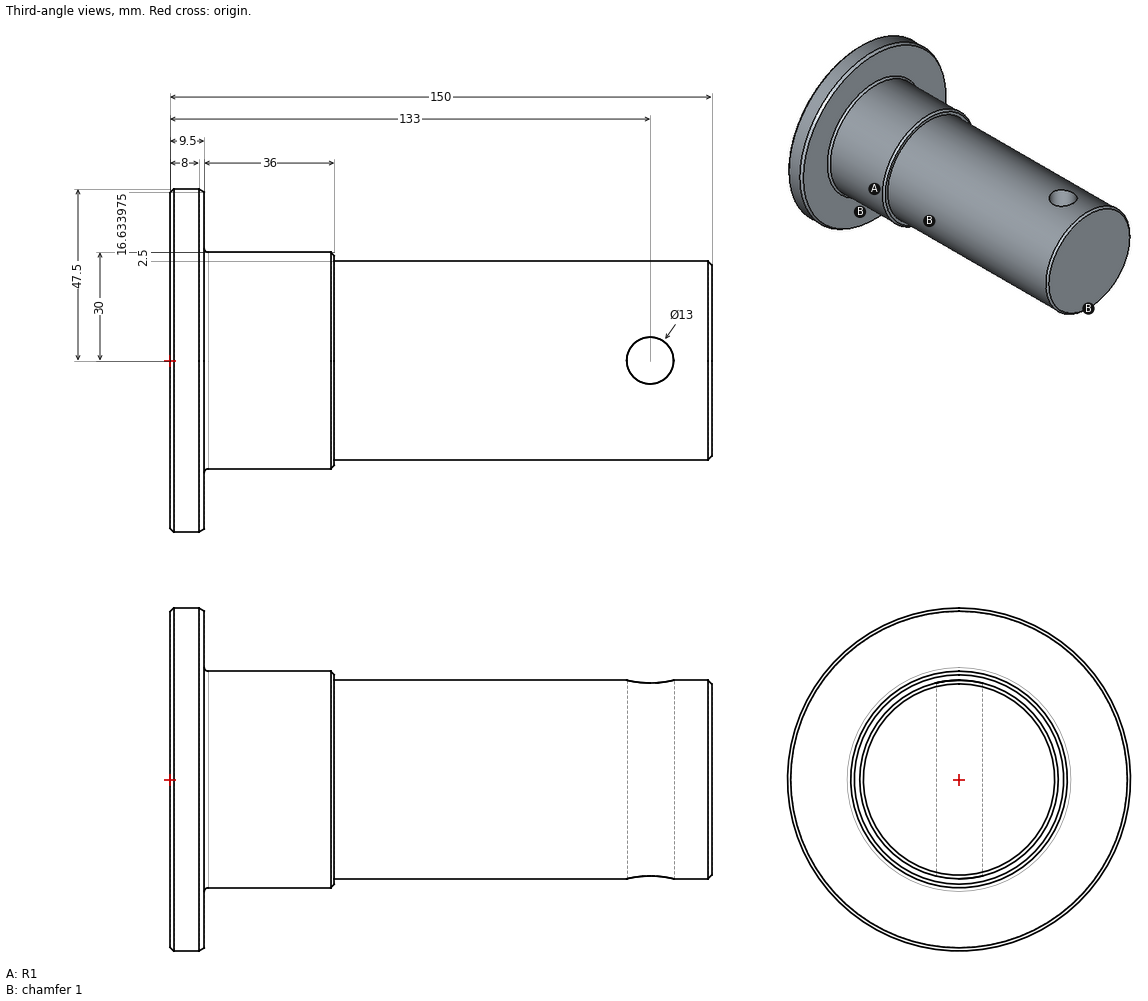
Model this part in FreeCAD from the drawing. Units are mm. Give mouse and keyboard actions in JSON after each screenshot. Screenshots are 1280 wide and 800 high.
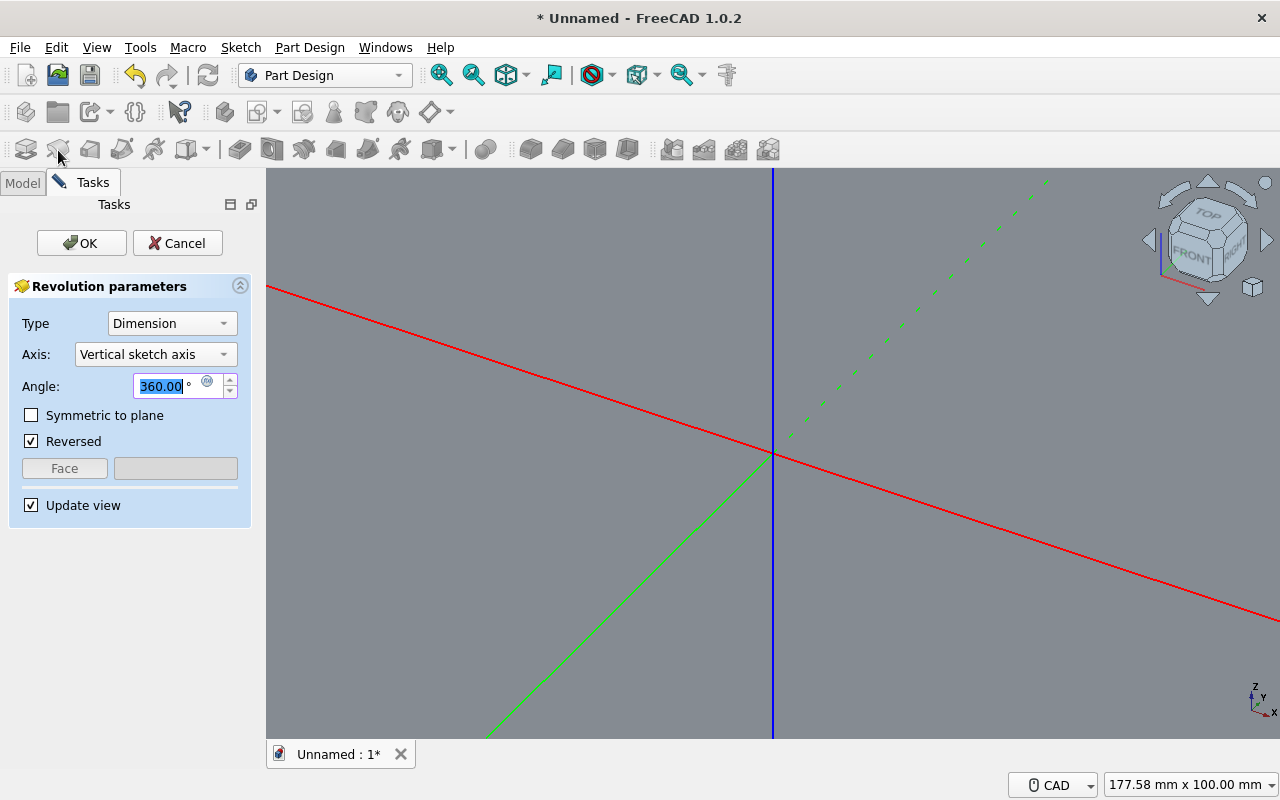
{"action": "left_click", "coordinate": [156, 354]}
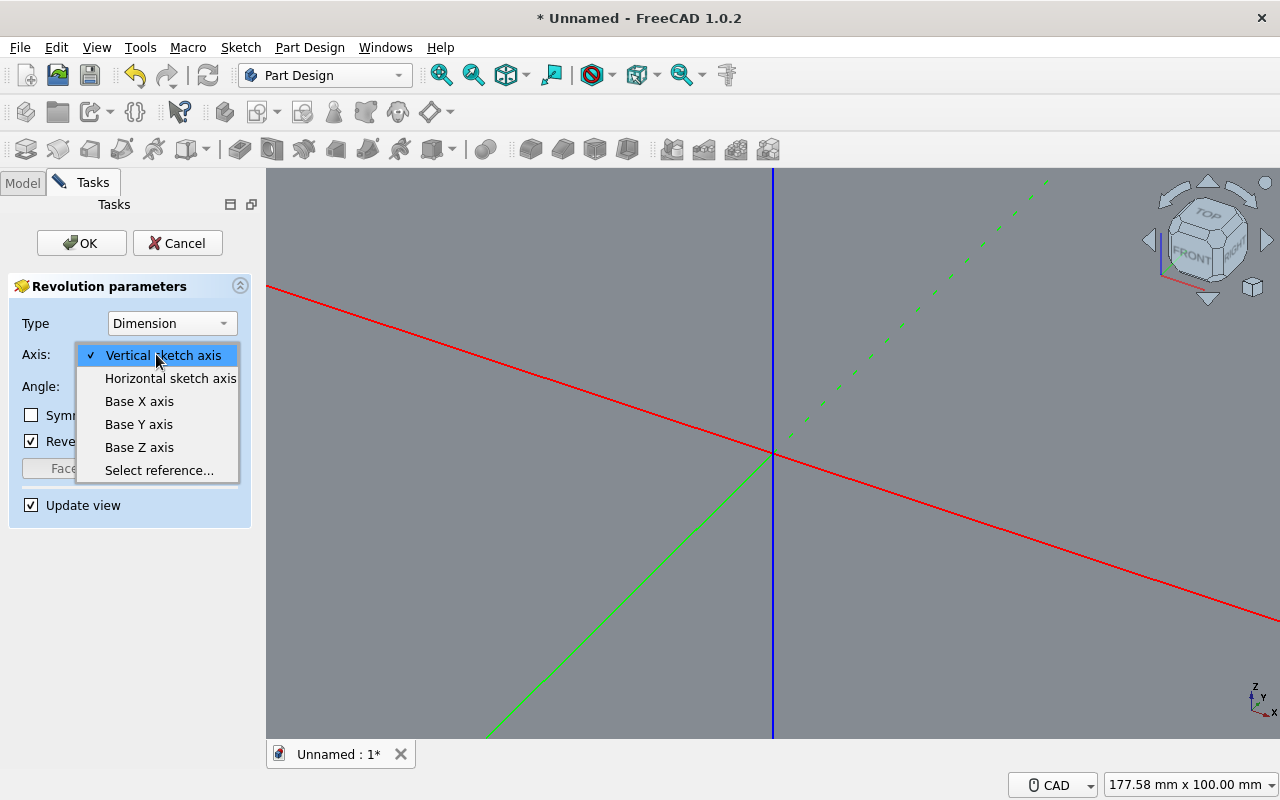
{"action": "left_click", "coordinate": [156, 378]}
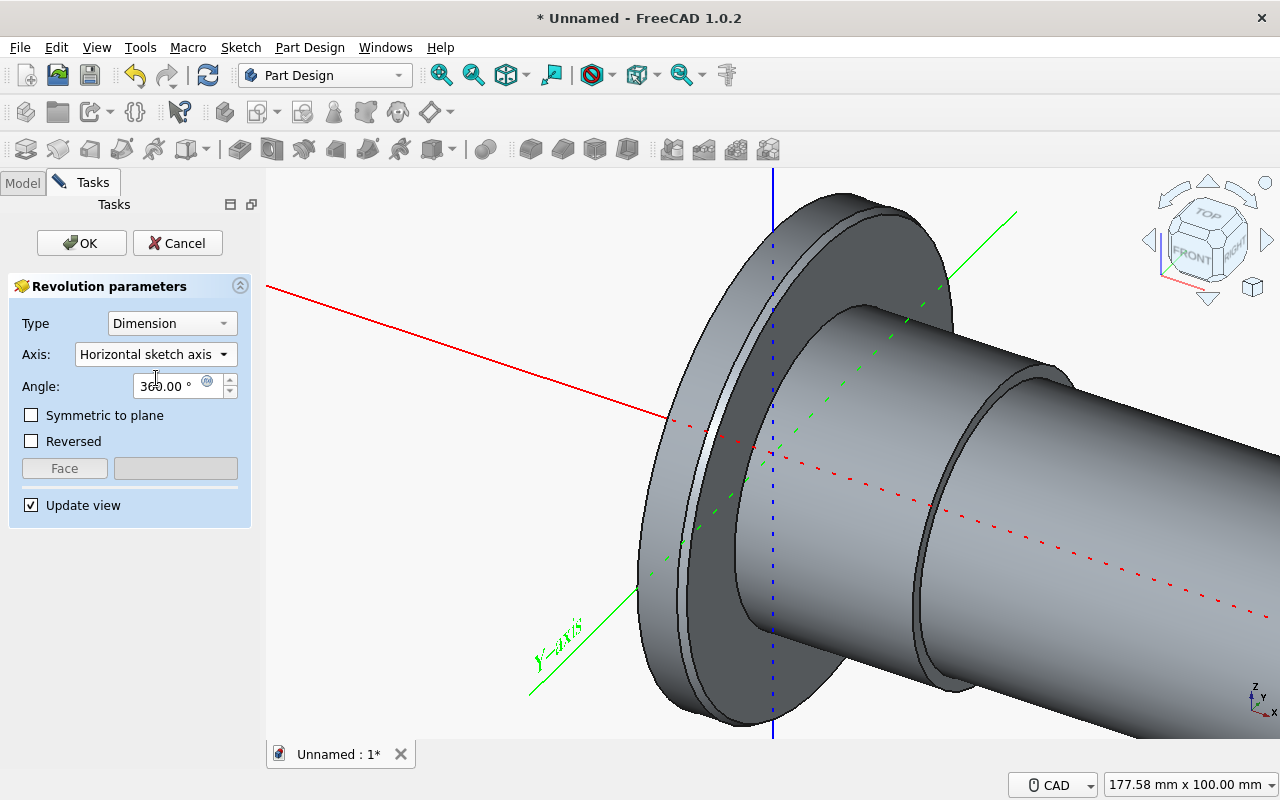
{"action": "left_click", "coordinate": [82, 243]}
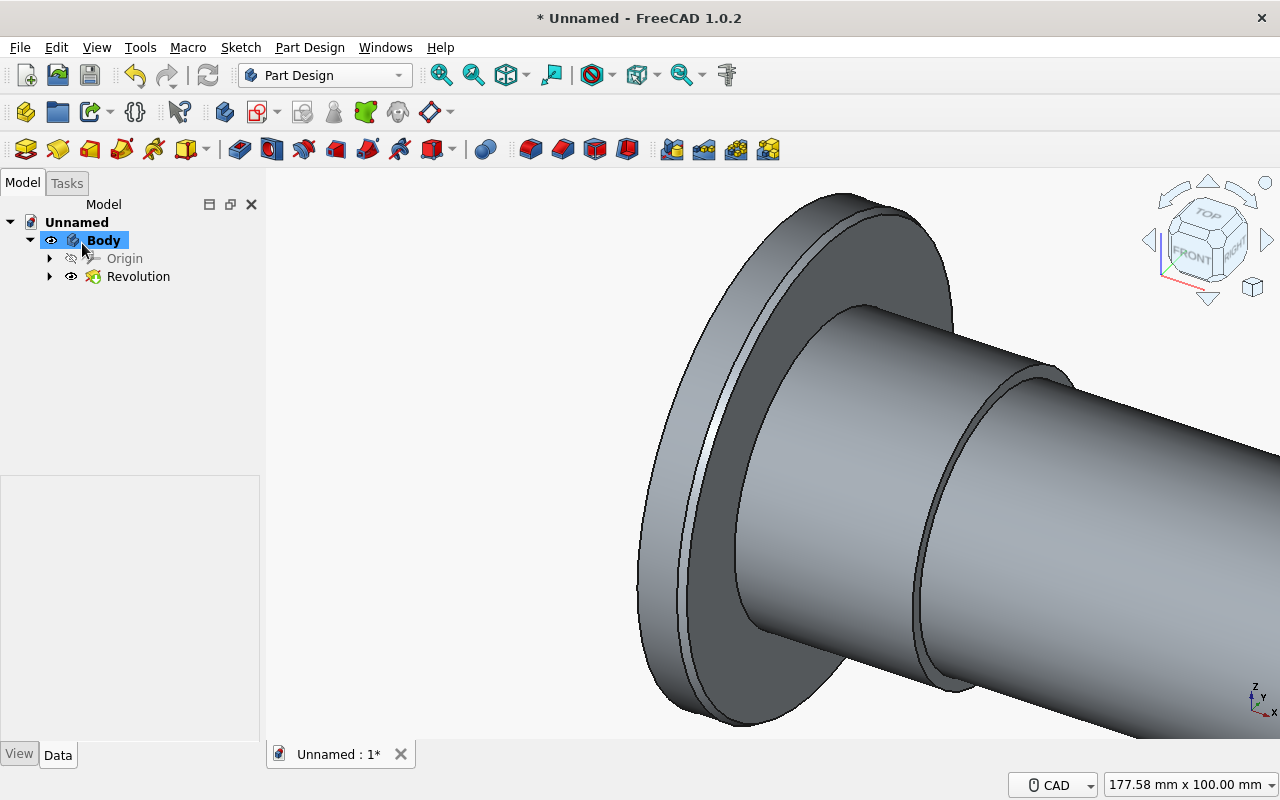
{"action": "key", "text": "v f"}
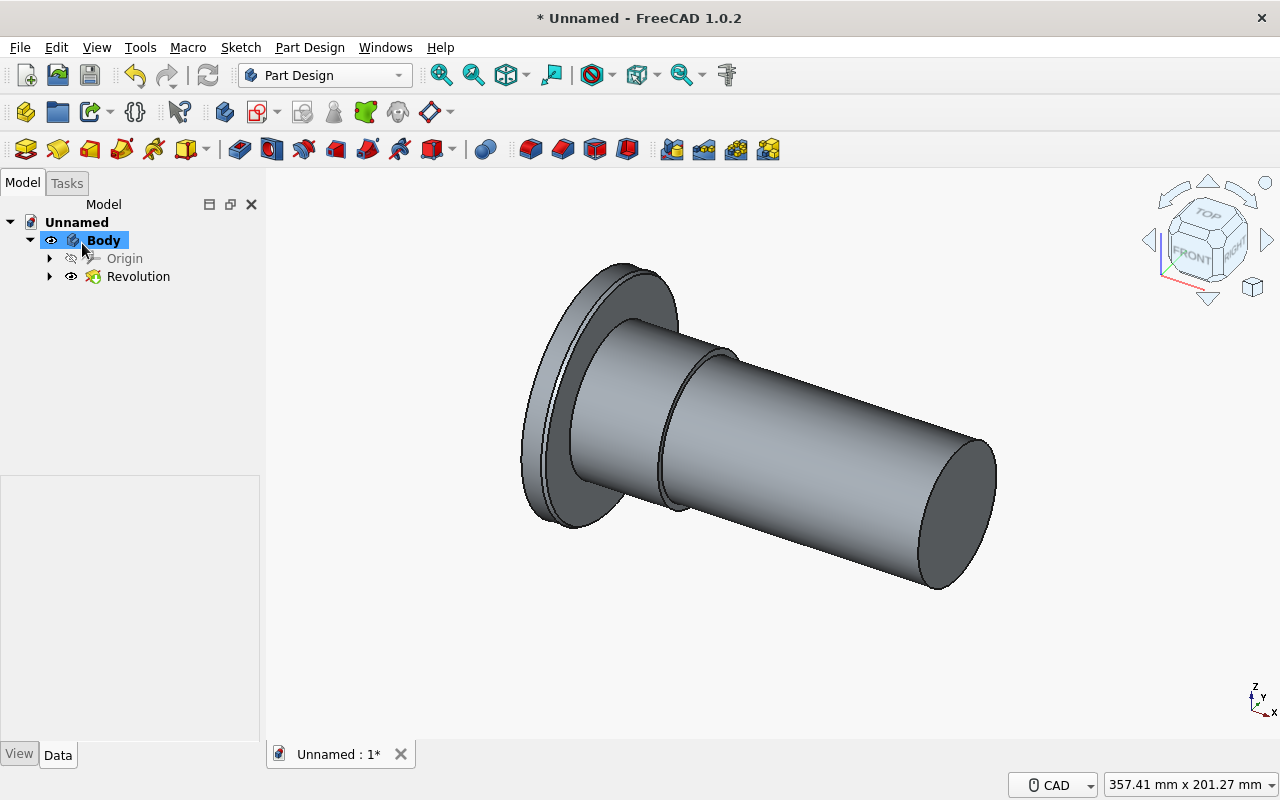
{"action": "key", "text": "0"}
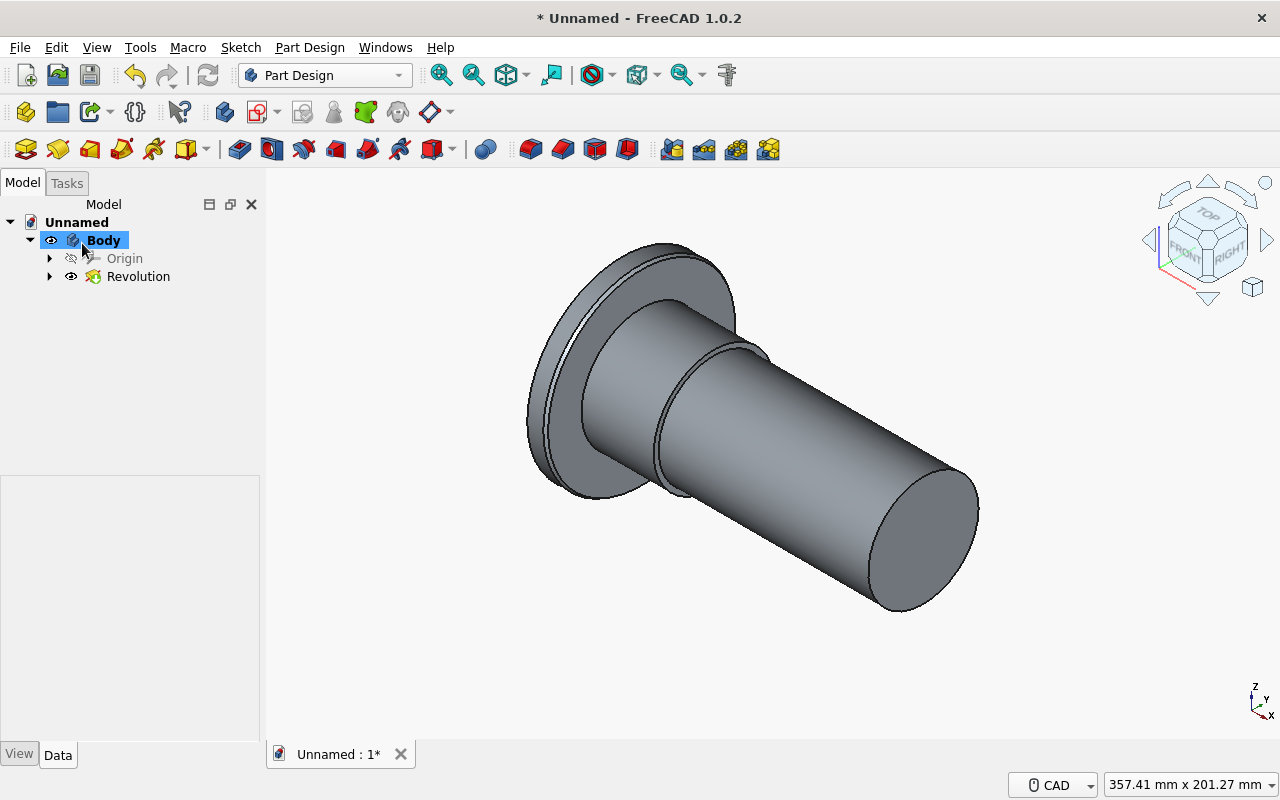
{"action": "key", "text": "2"}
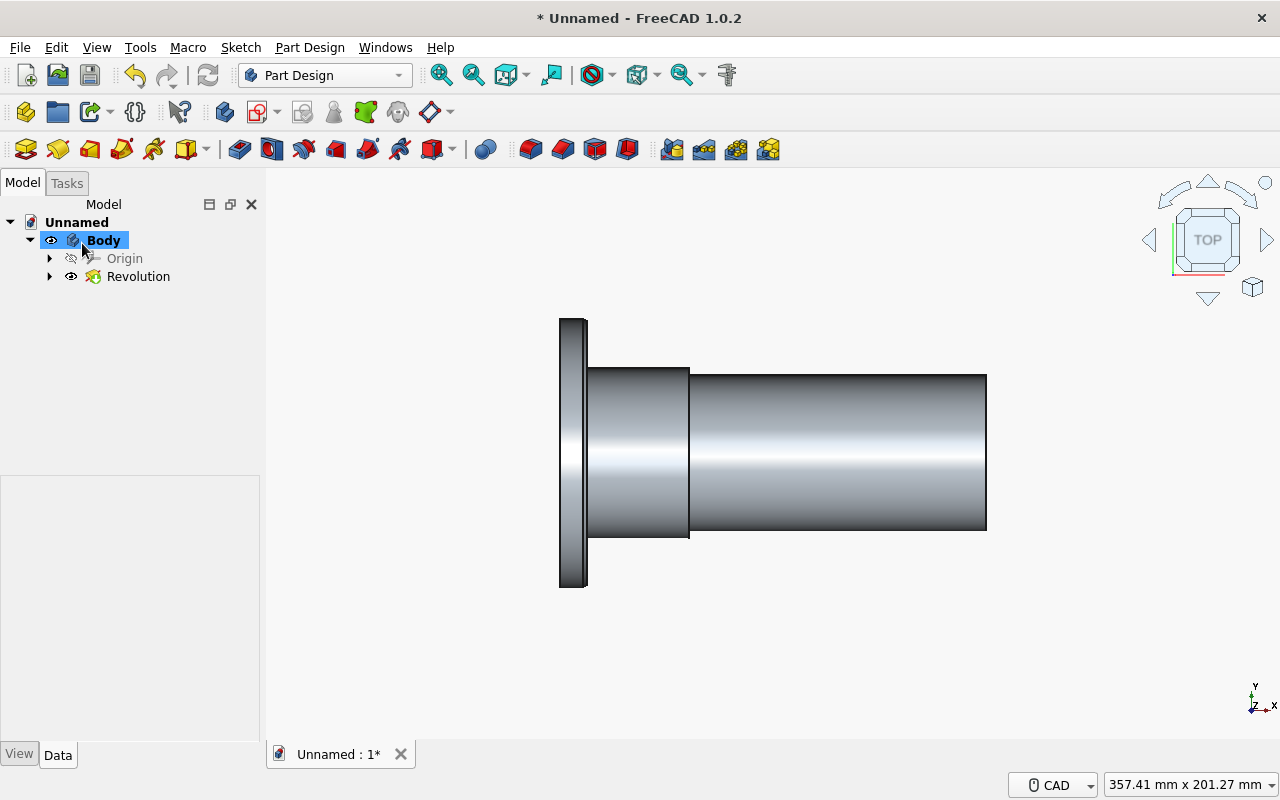
{"action": "key", "text": "1"}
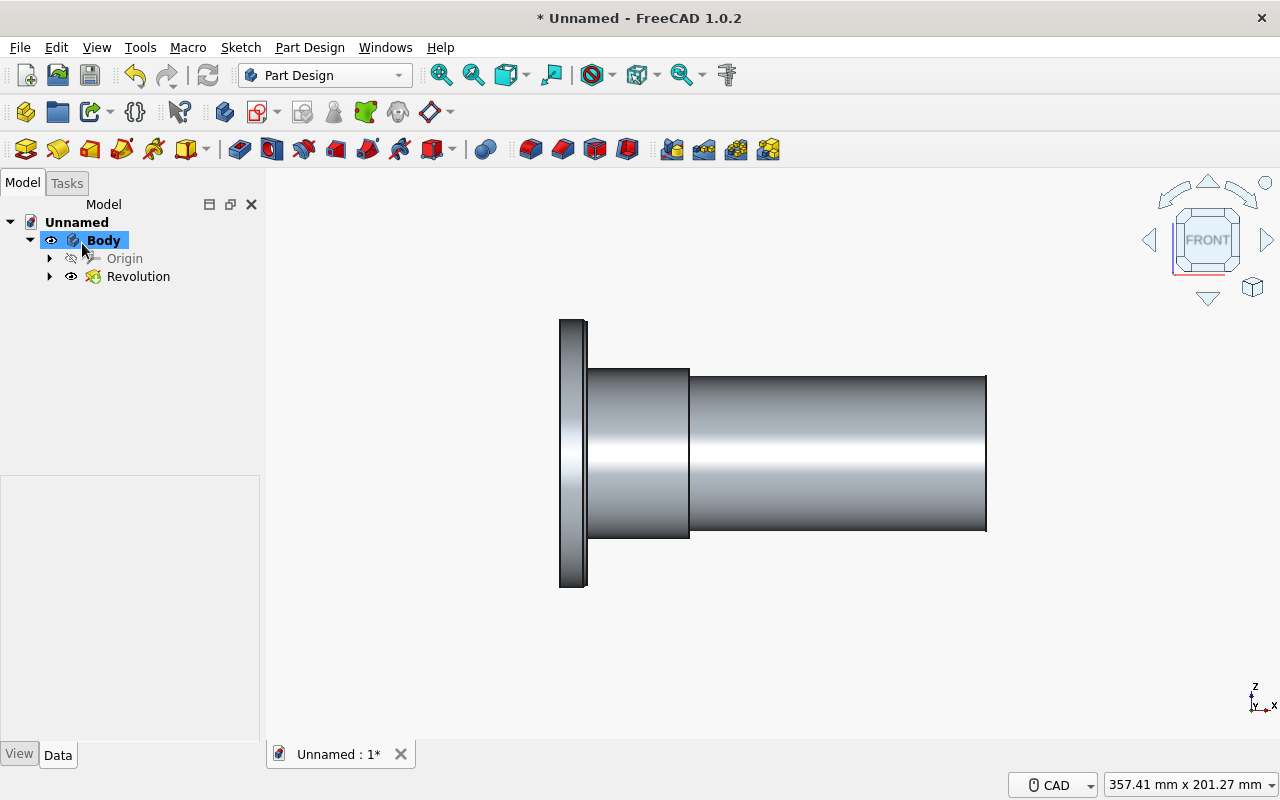
{"action": "key", "text": "3"}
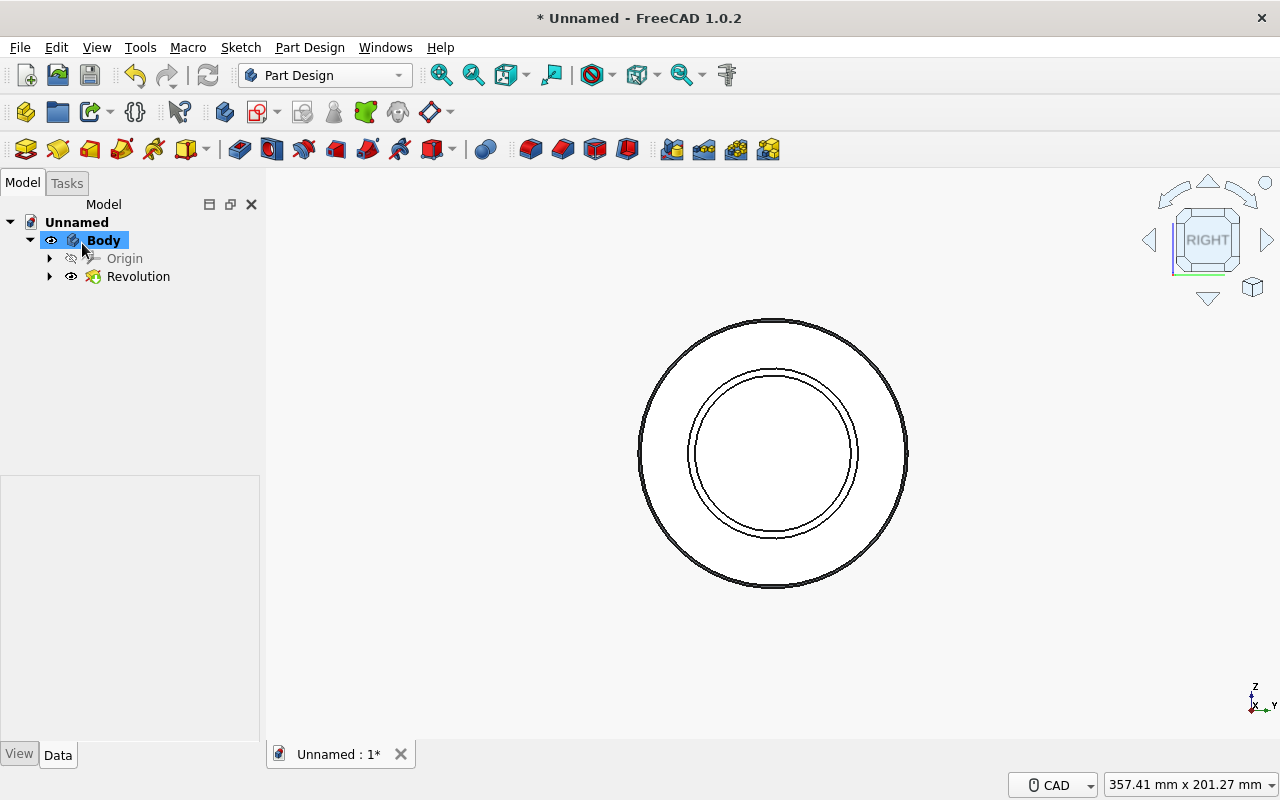
{"action": "key", "text": "5"}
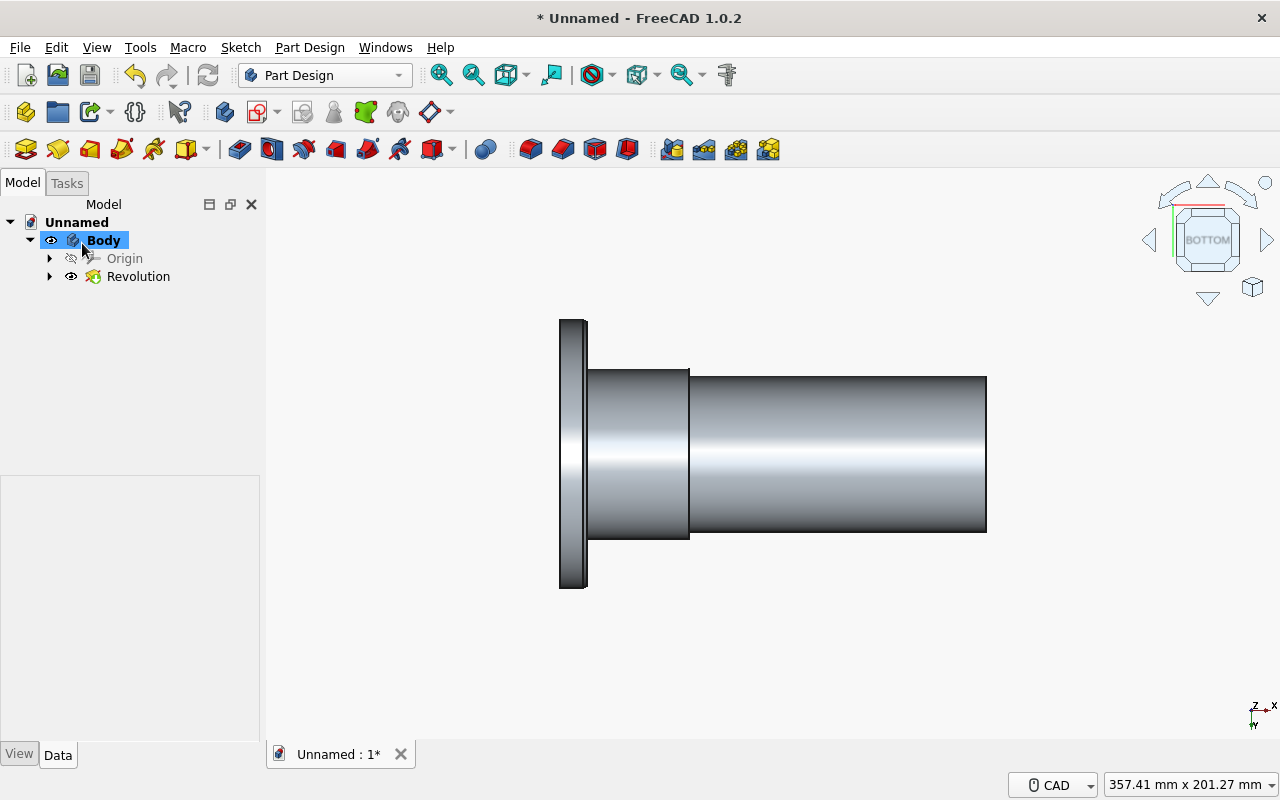
{"action": "key", "text": "4"}